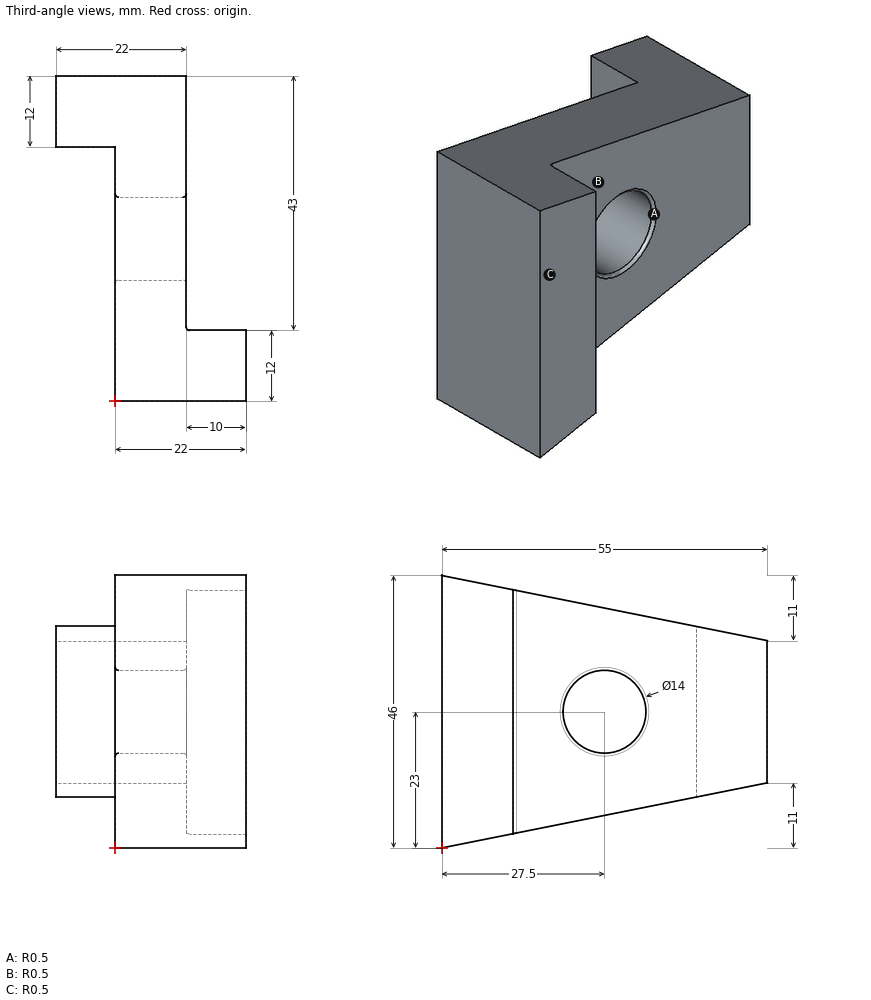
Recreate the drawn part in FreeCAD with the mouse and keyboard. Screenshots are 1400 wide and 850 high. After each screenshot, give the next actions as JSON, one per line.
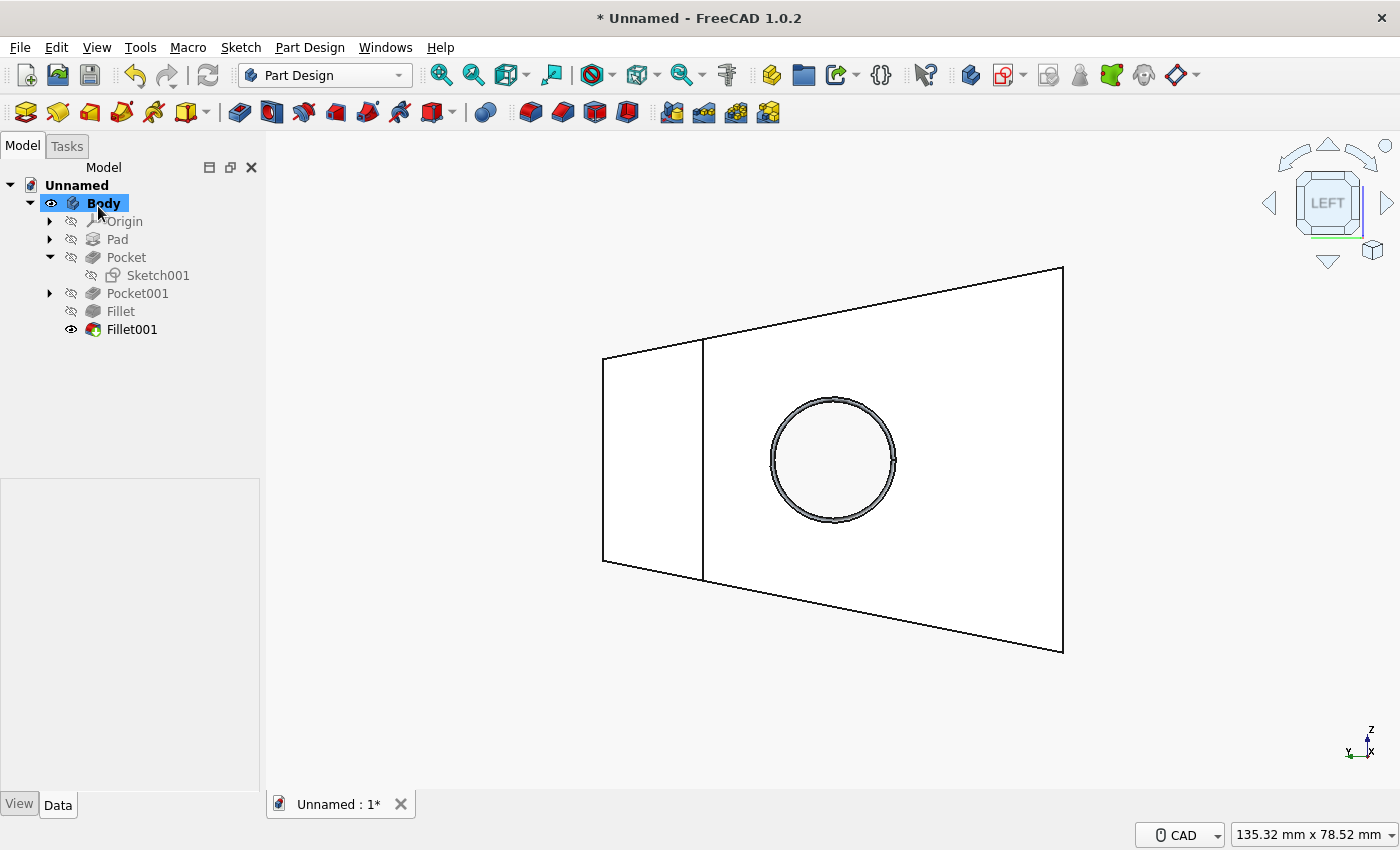
{"action": "key", "text": "0"}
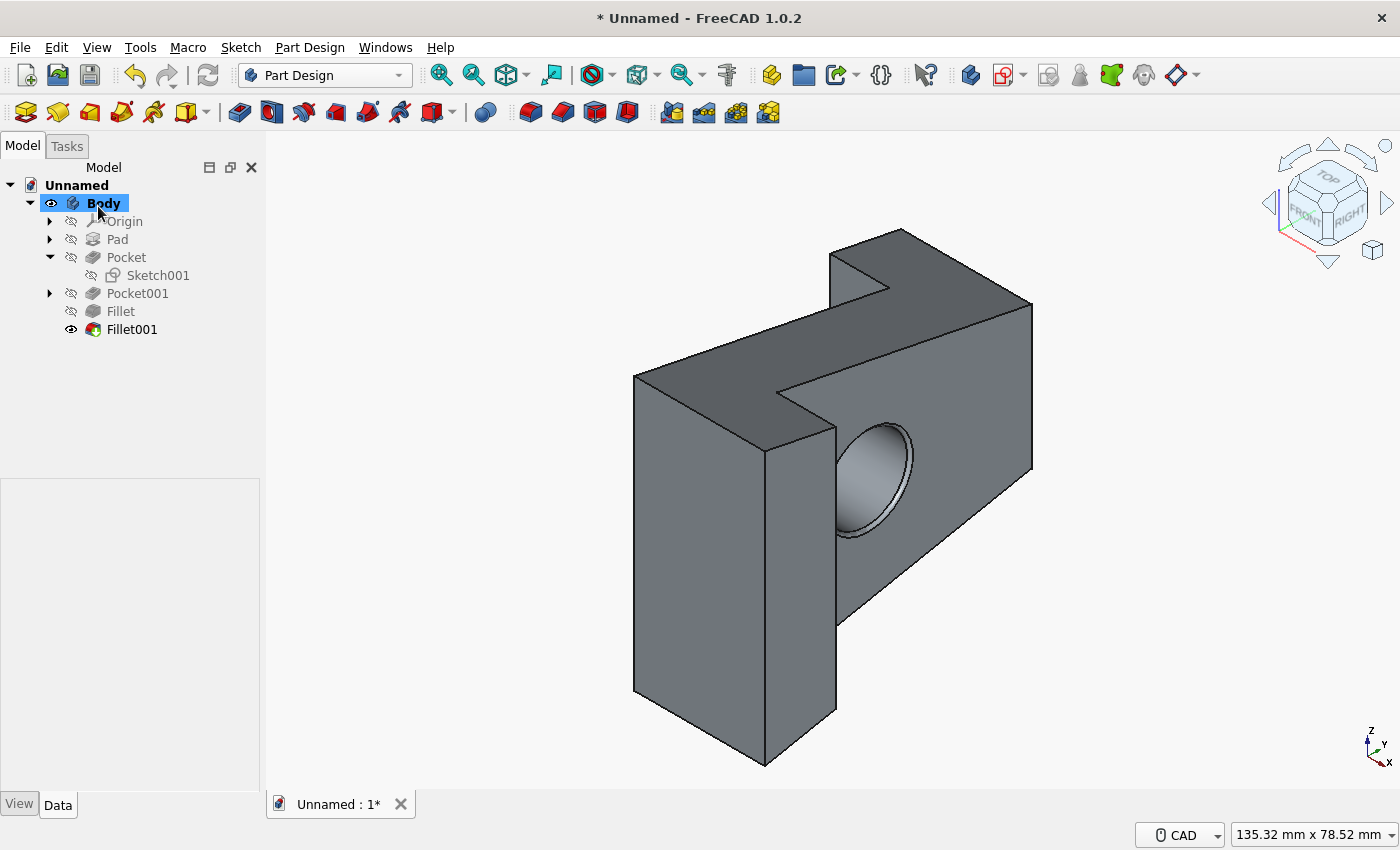
{"action": "key", "text": "2"}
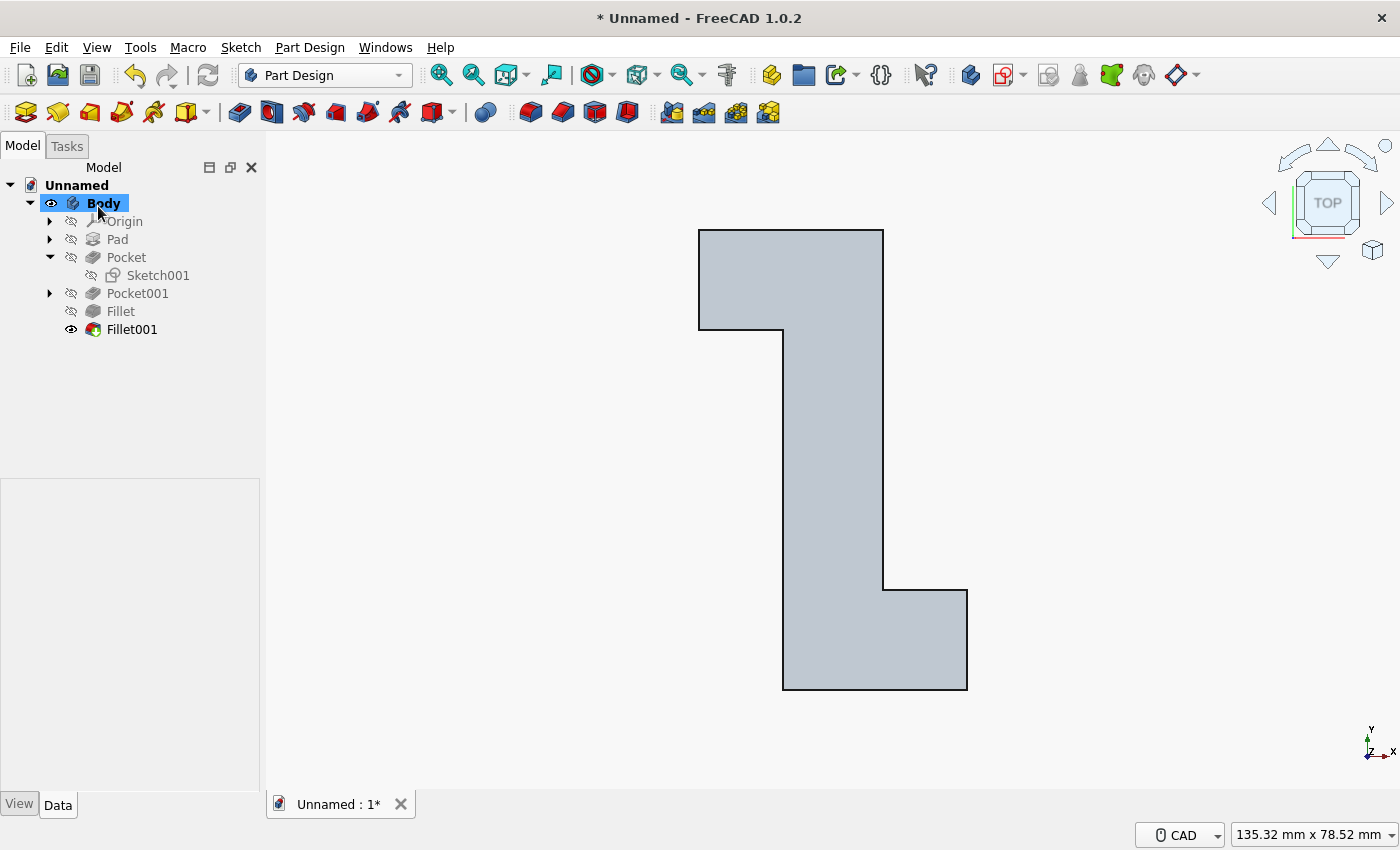
{"action": "key", "text": "1"}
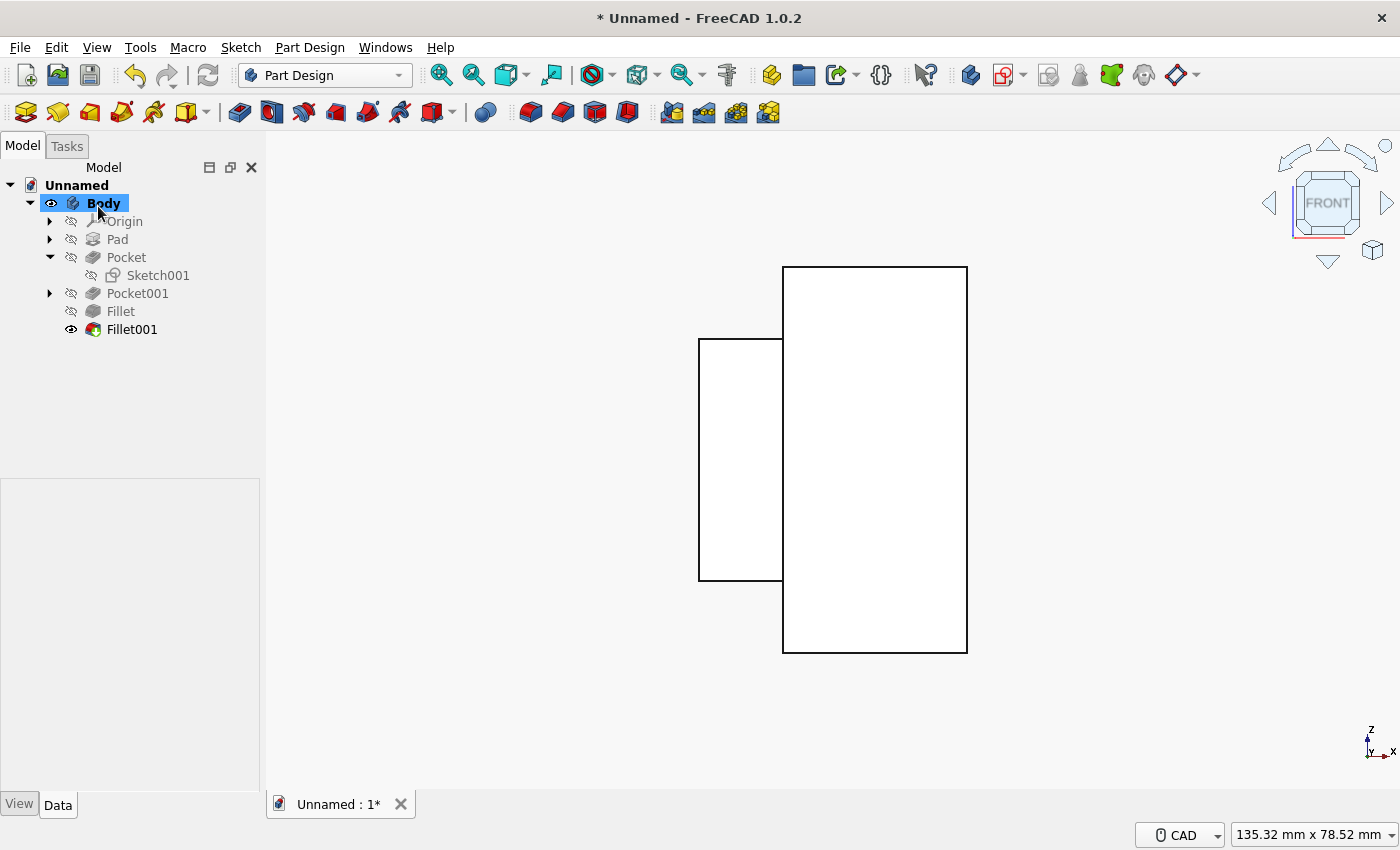
{"action": "key", "text": "3"}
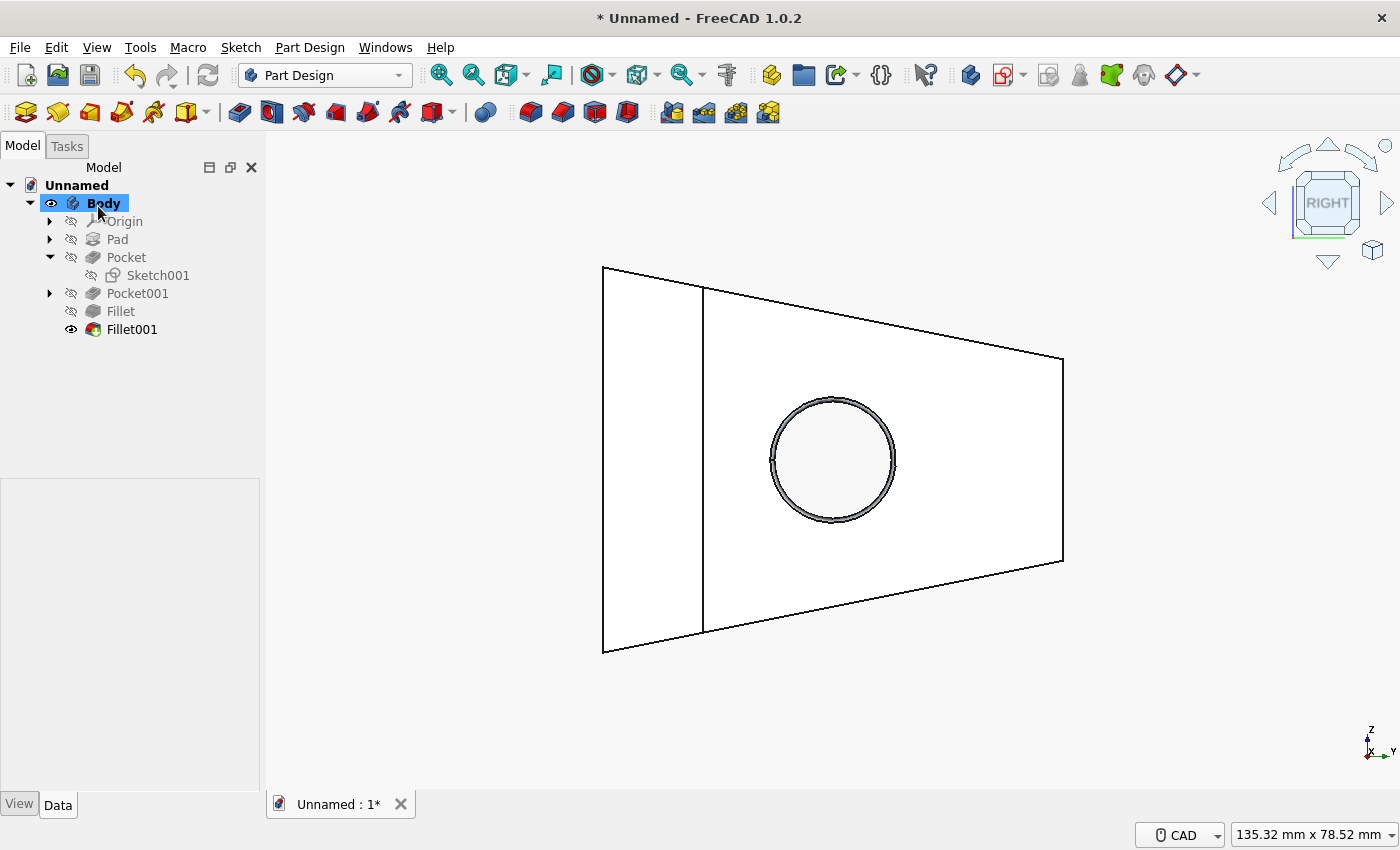
{"action": "key", "text": "5"}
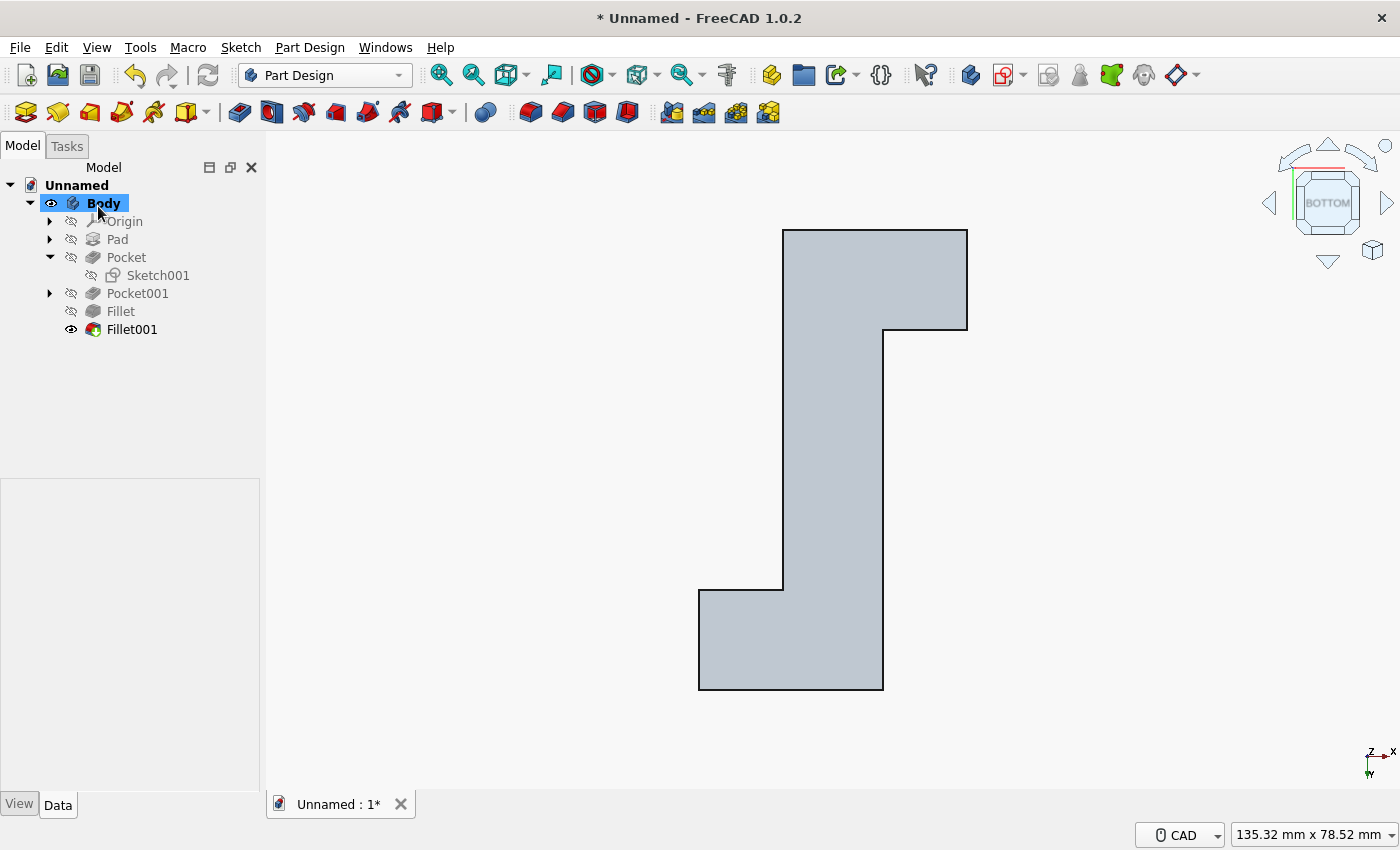
{"action": "key", "text": "4"}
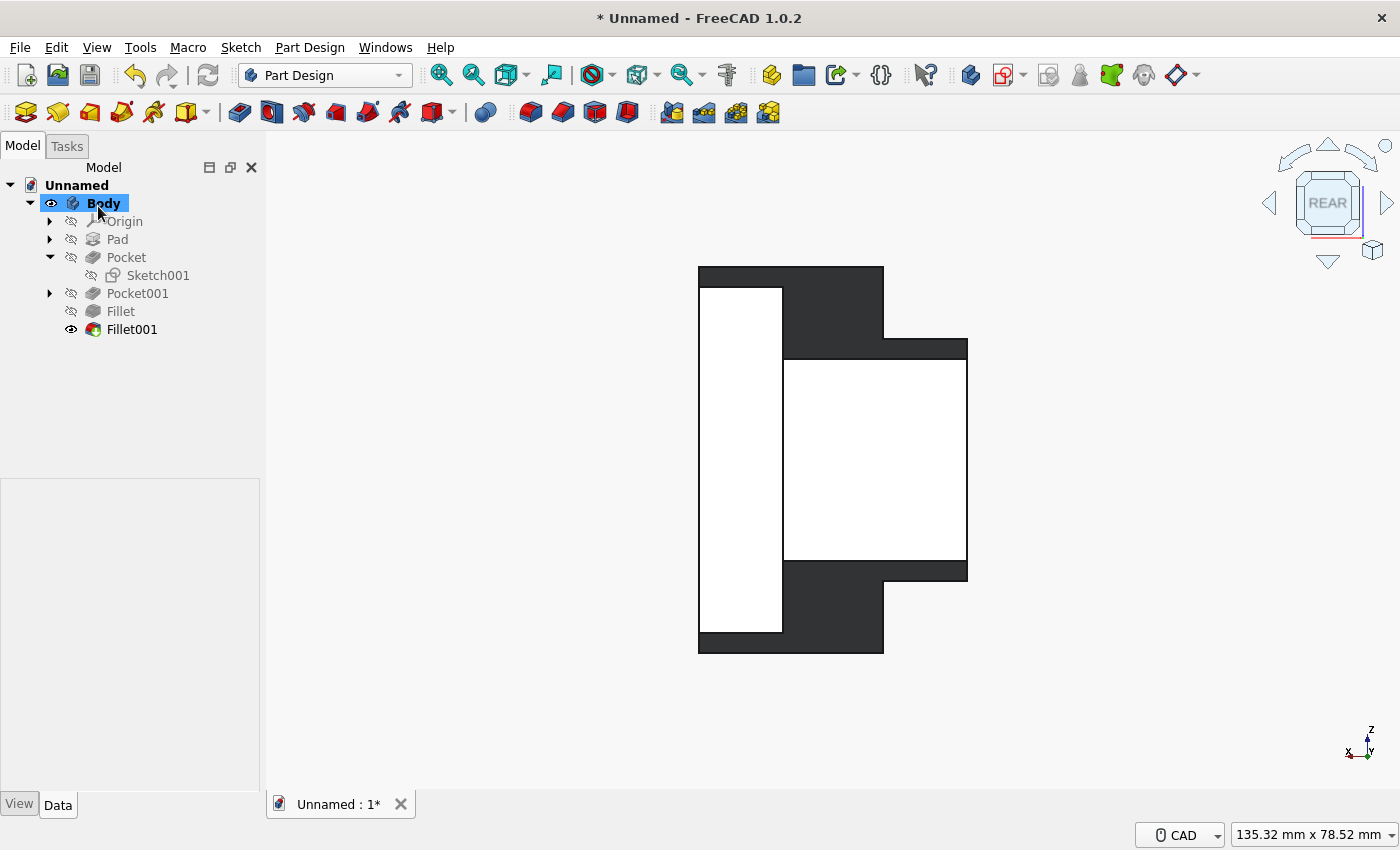
{"action": "key", "text": "6"}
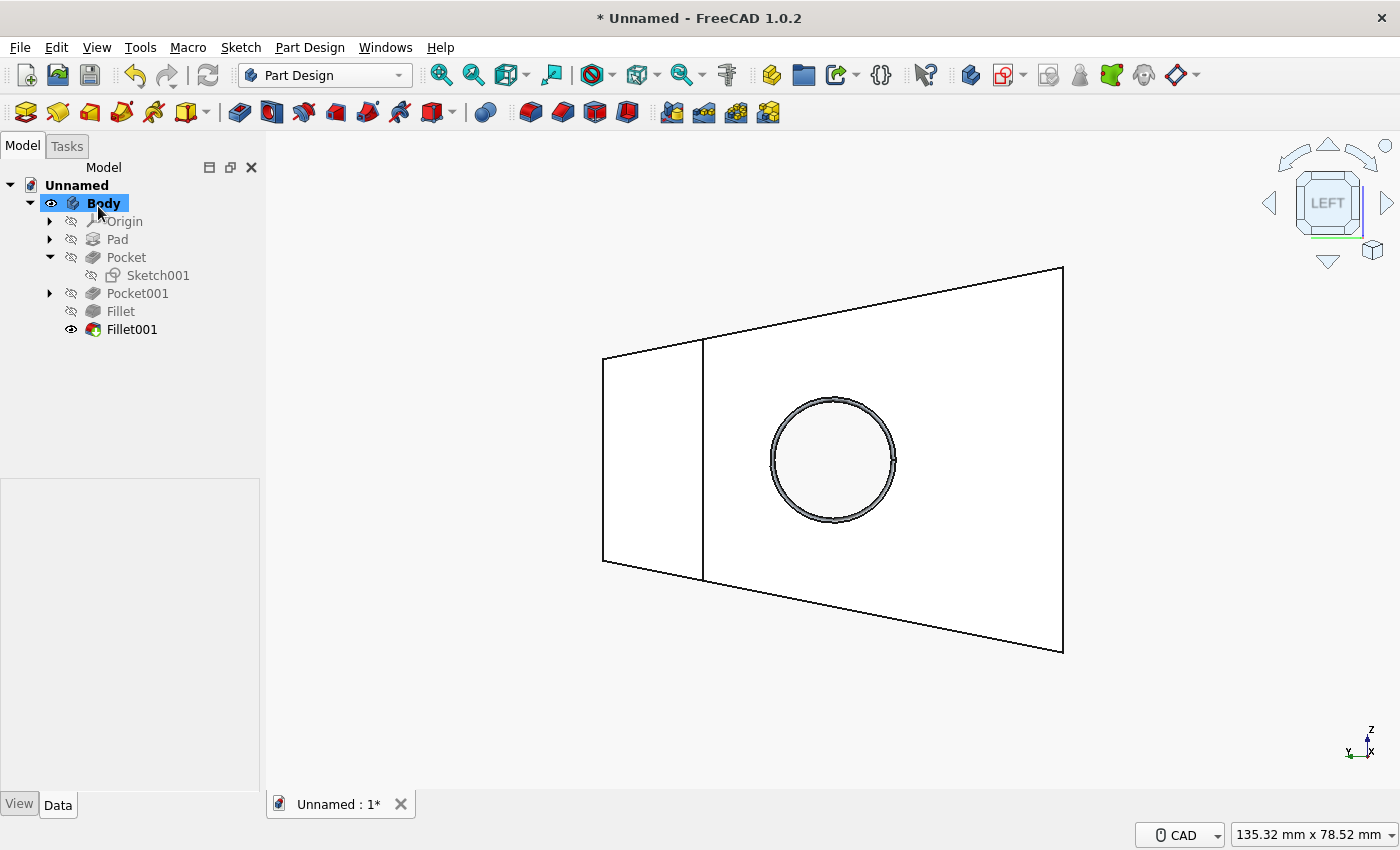
{"action": "key", "text": "v 3"}